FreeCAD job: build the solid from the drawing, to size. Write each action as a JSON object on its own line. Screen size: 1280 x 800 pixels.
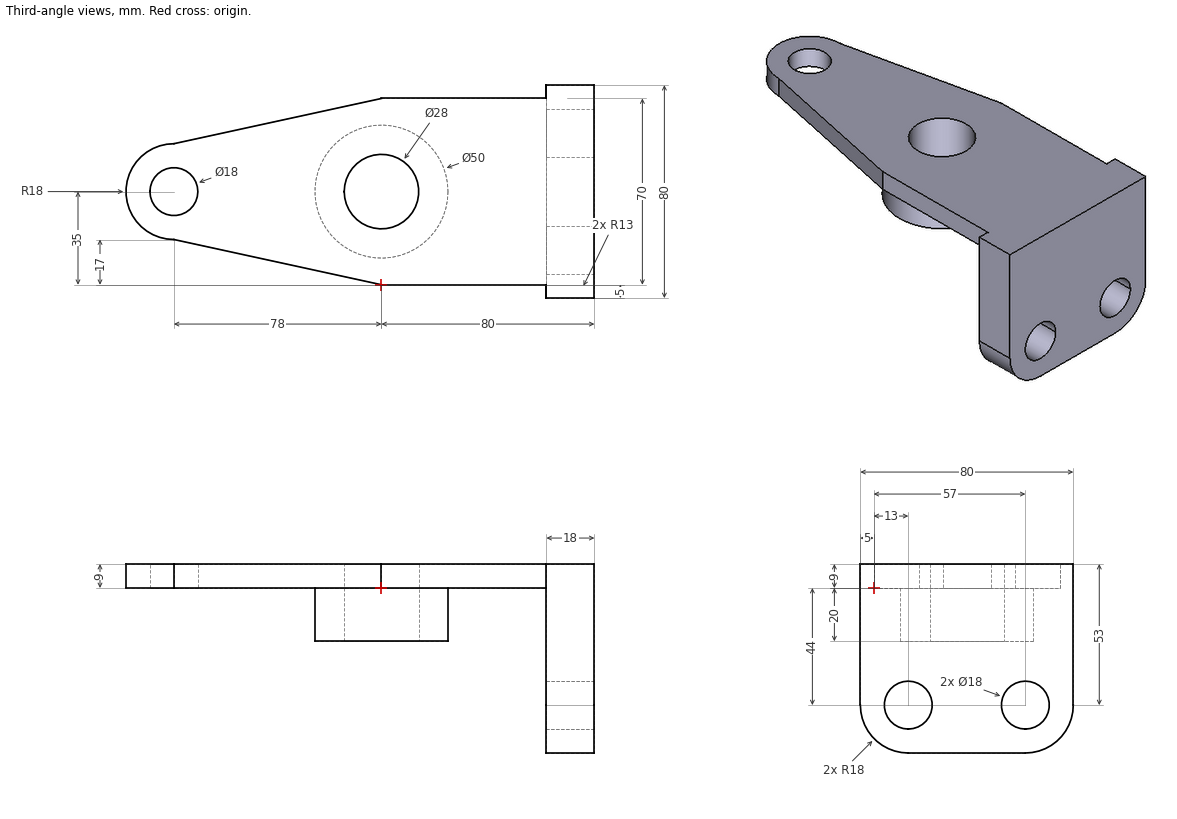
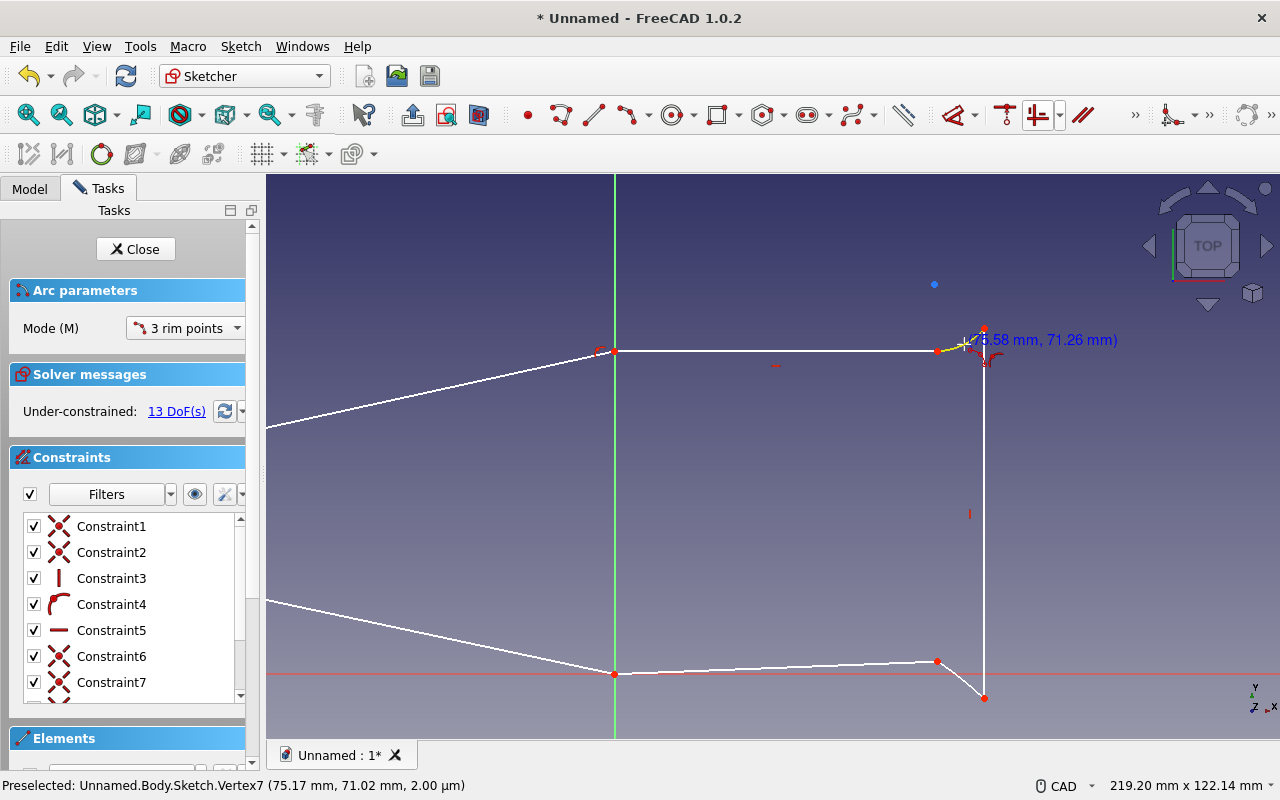
{"action": "left_click", "coordinate": [489, 402]}
{"action": "left_click", "coordinate": [489, 514]}
{"action": "left_click", "coordinate": [432, 457]}
{"action": "key", "text": "Escape"}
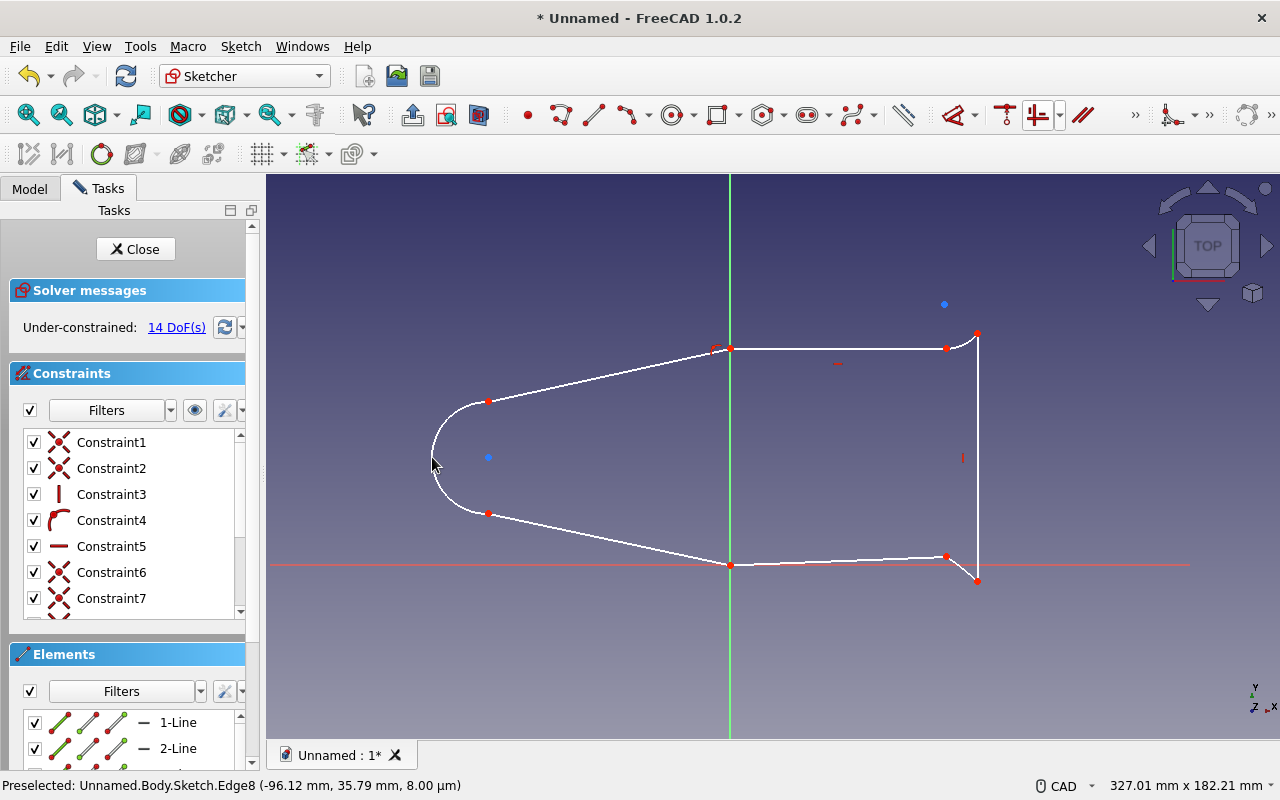
{"action": "left_click", "coordinate": [795, 563]}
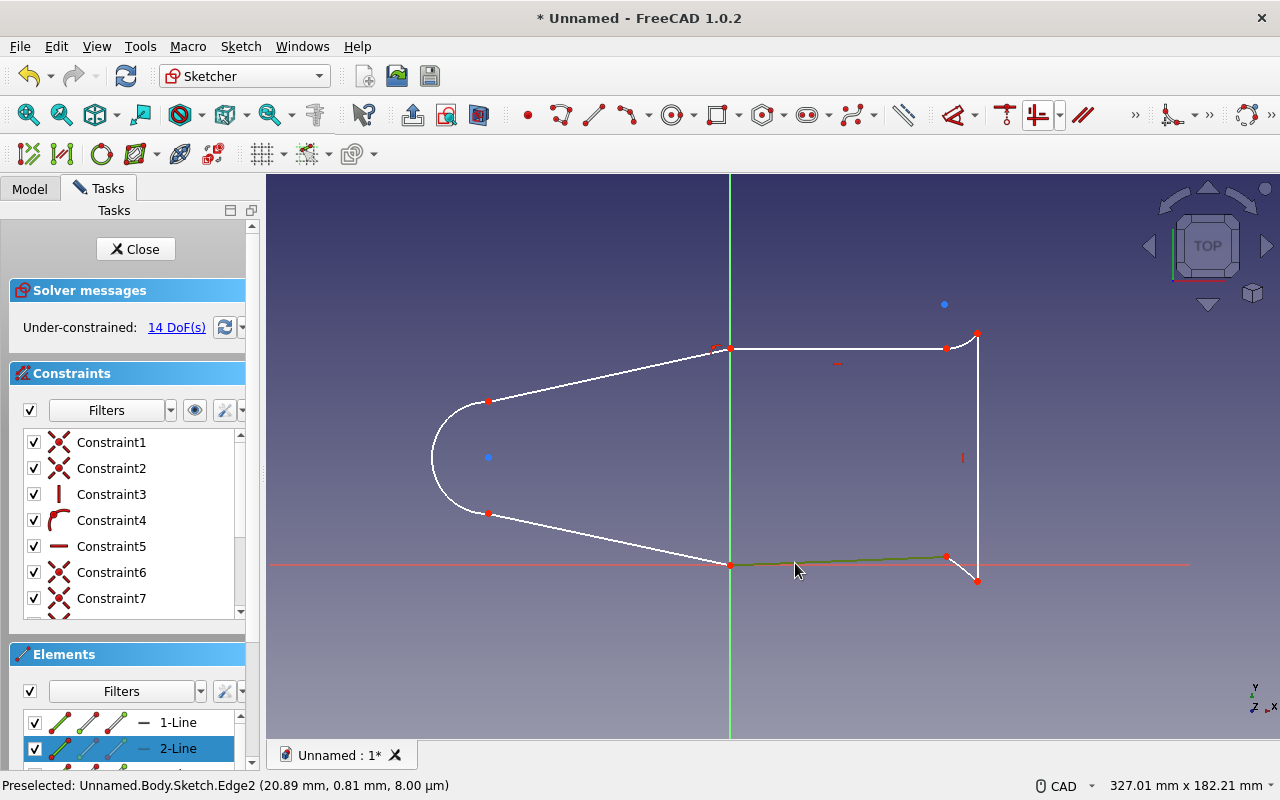
{"action": "left_click", "coordinate": [957, 564]}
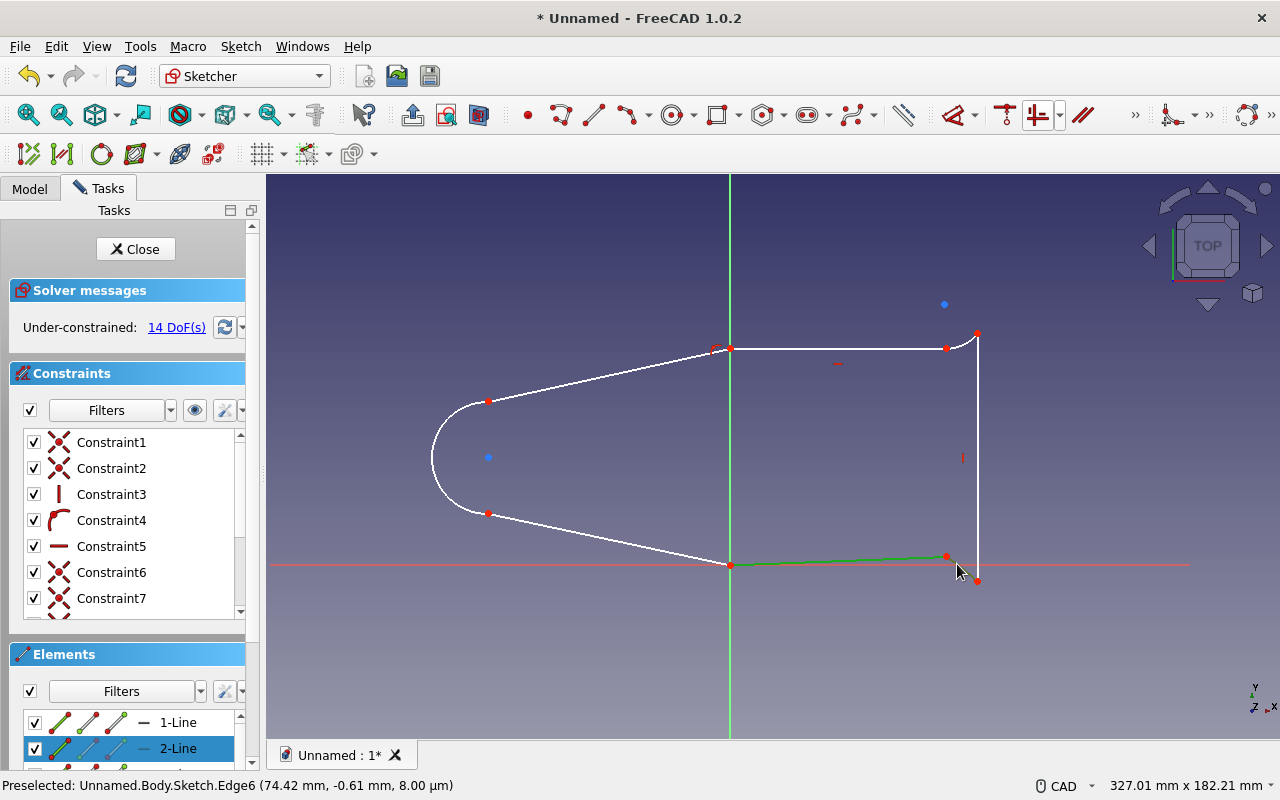
{"action": "key", "text": "t"}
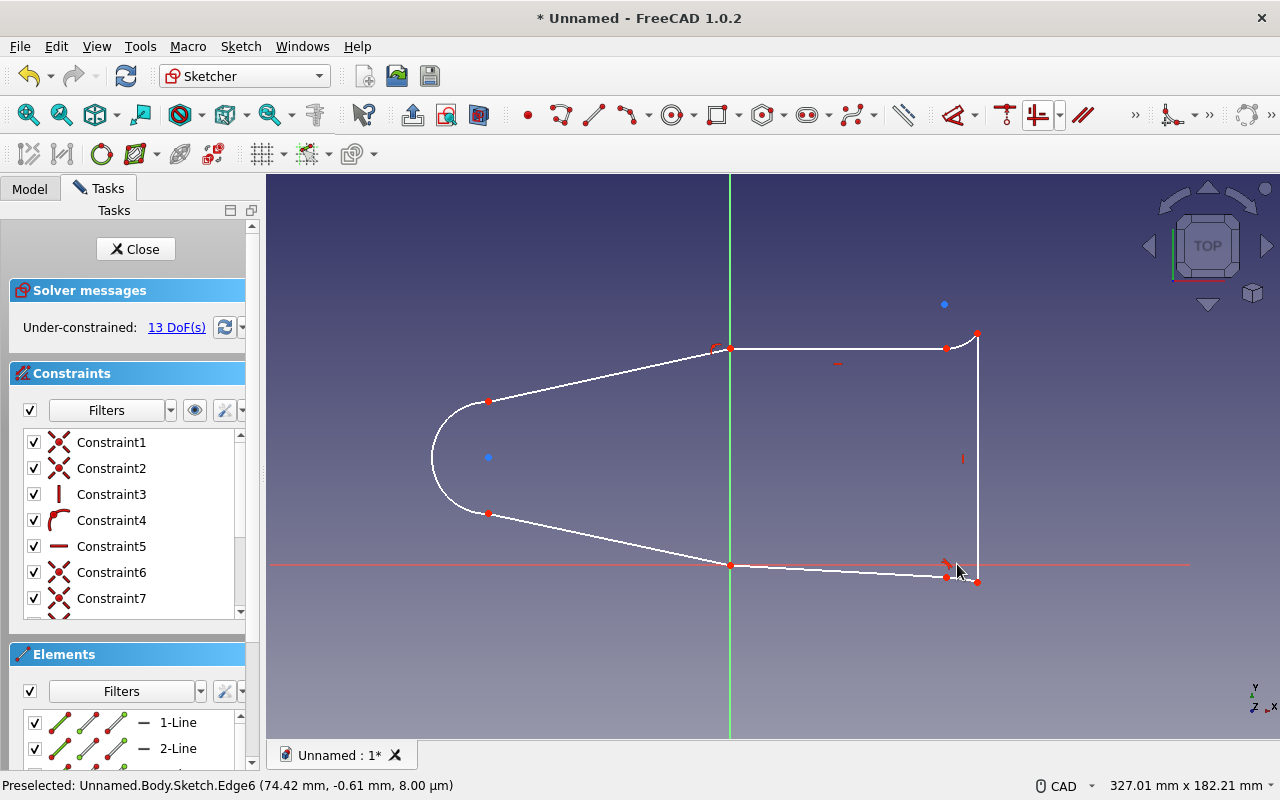
{"action": "left_click", "coordinate": [882, 349]}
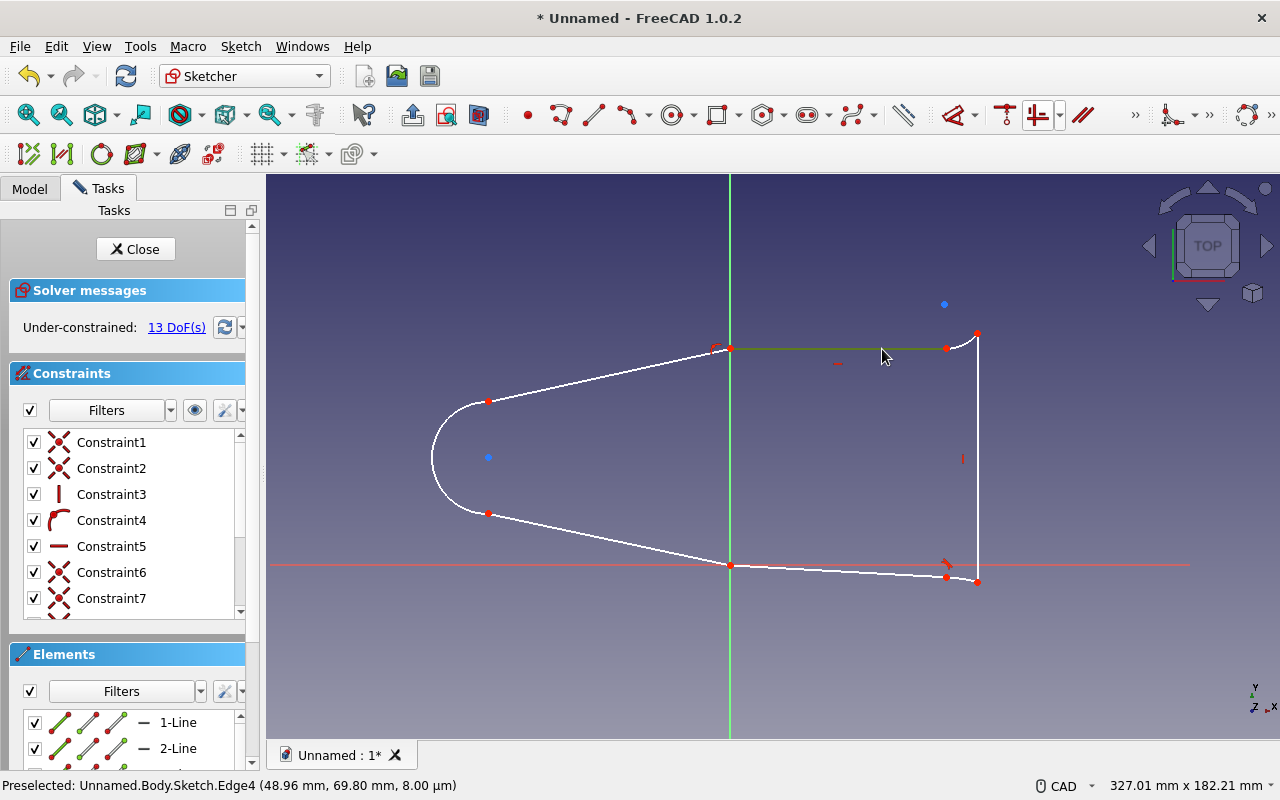
{"action": "scroll", "coordinate": [957, 347], "scroll_direction": "up", "scroll_amount": 2}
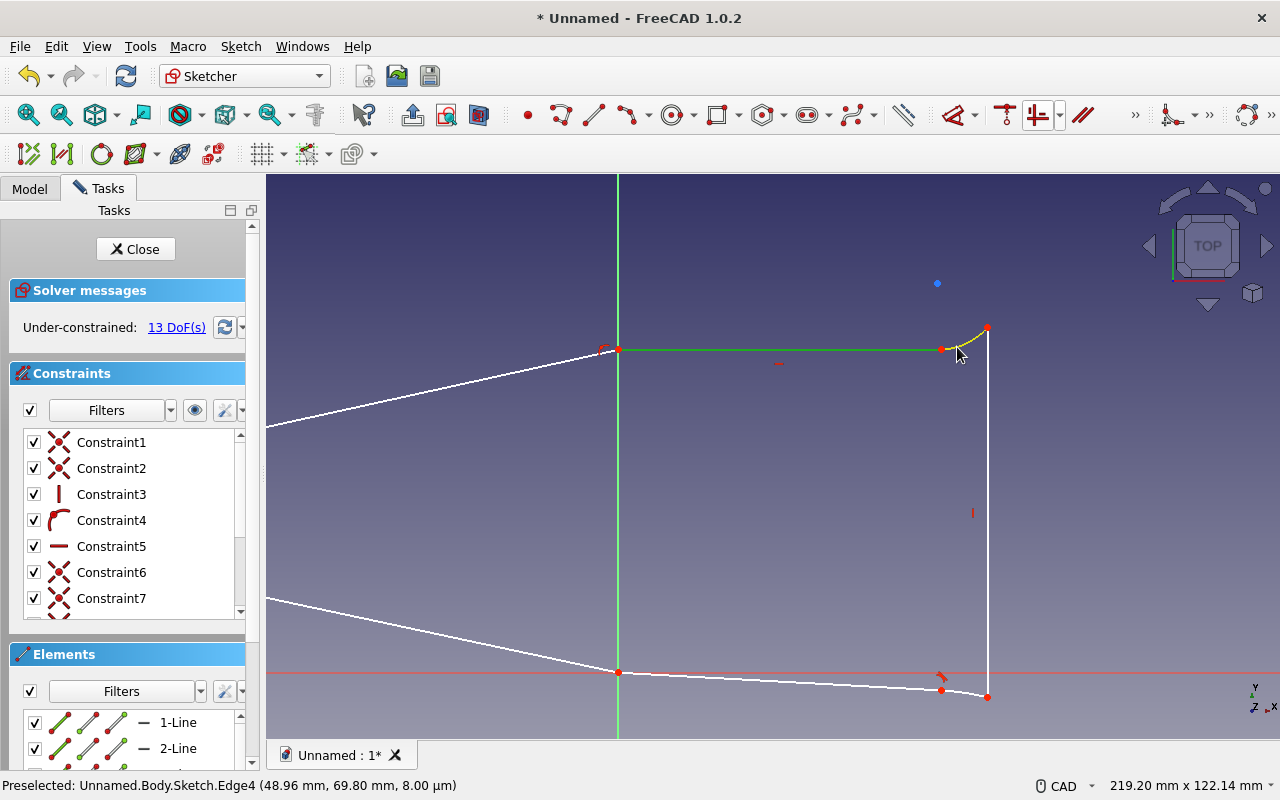
{"action": "left_click", "coordinate": [957, 347]}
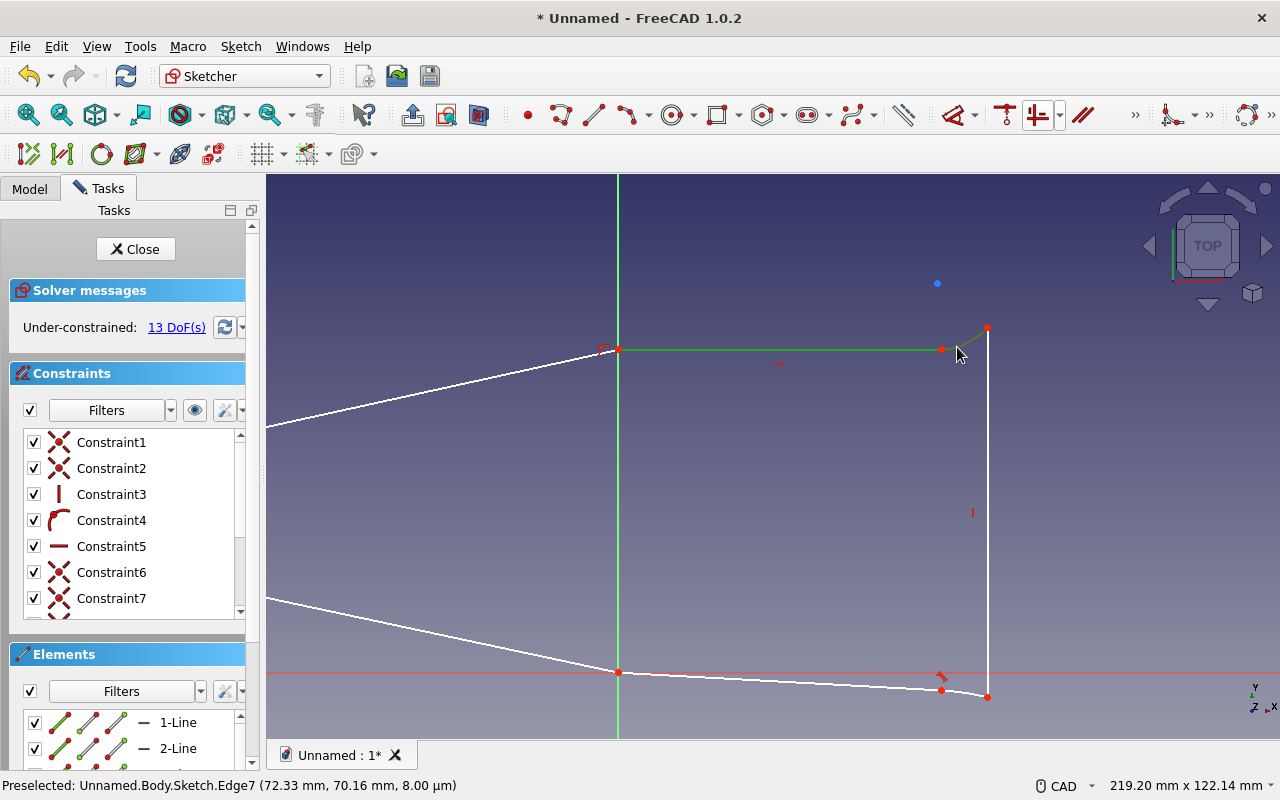
{"action": "key", "text": "t"}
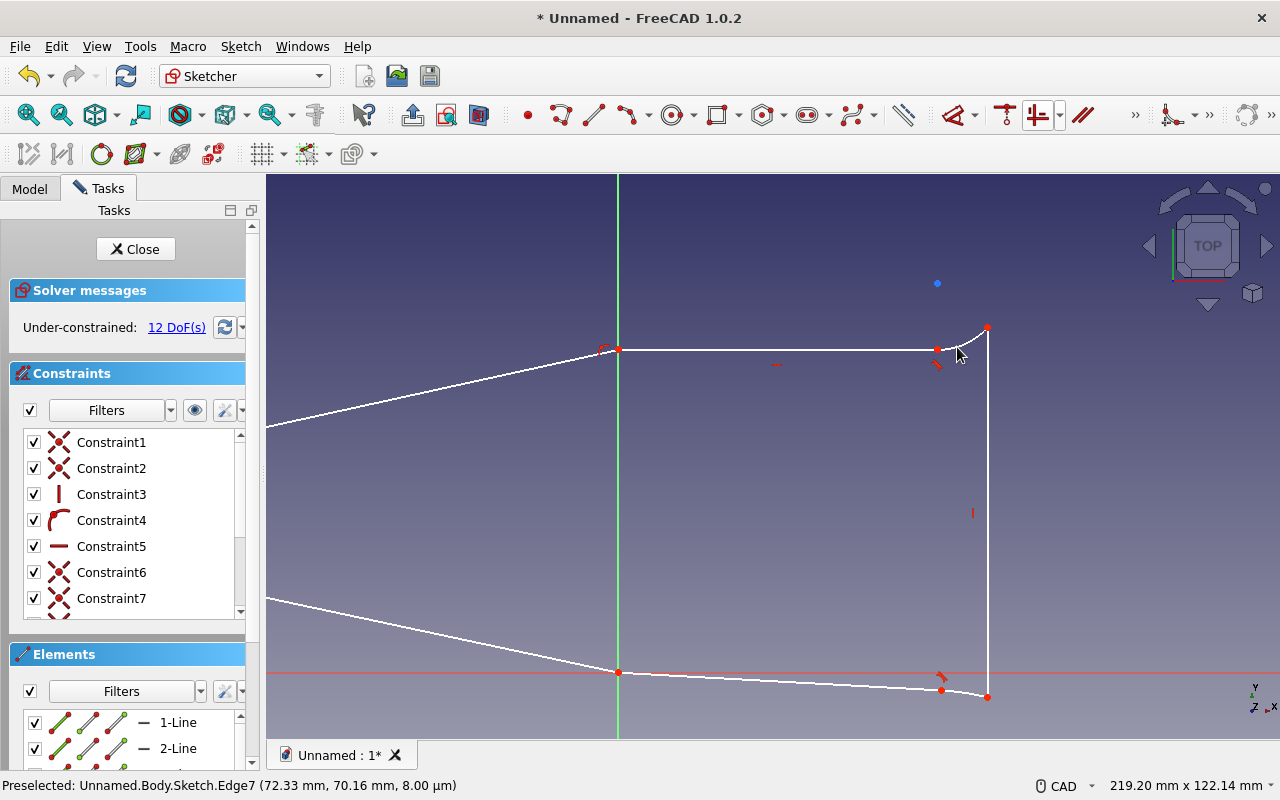
{"action": "left_click", "coordinate": [844, 685]}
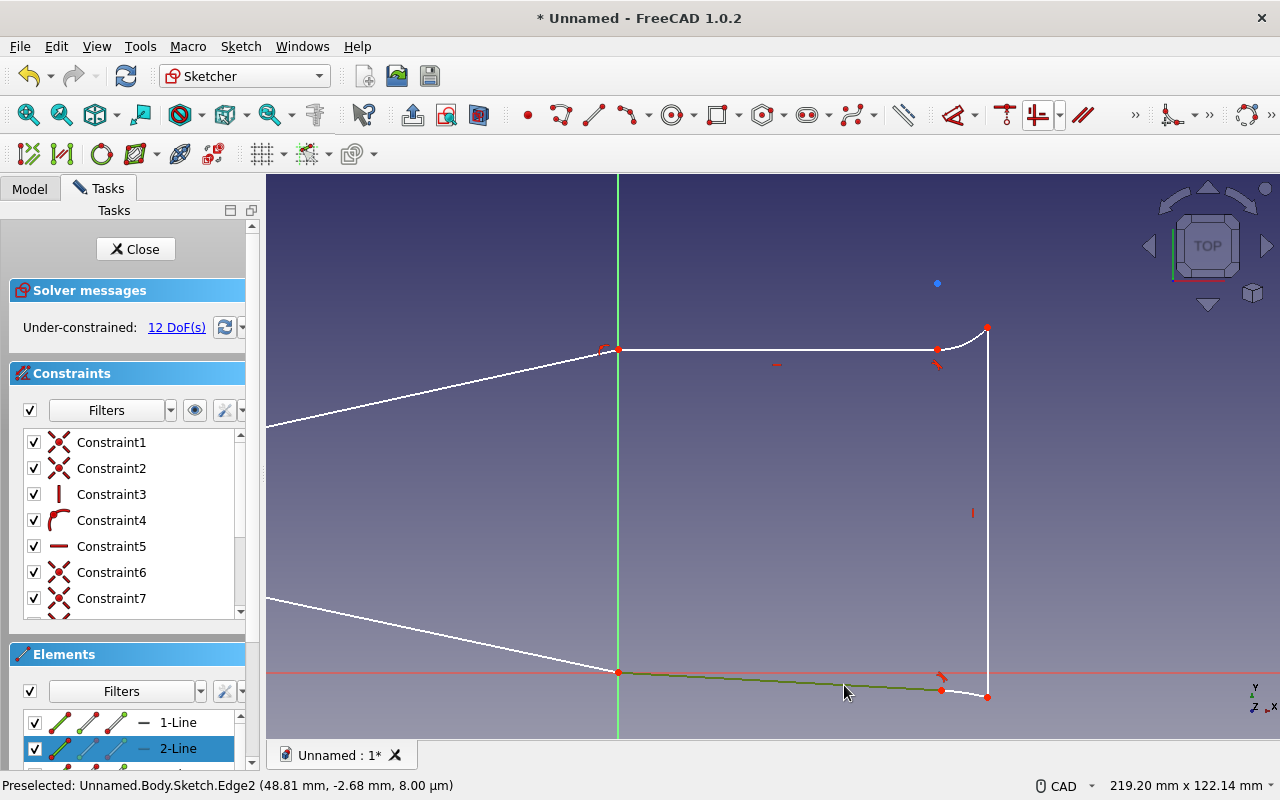
{"action": "left_click", "coordinate": [1060, 116]}